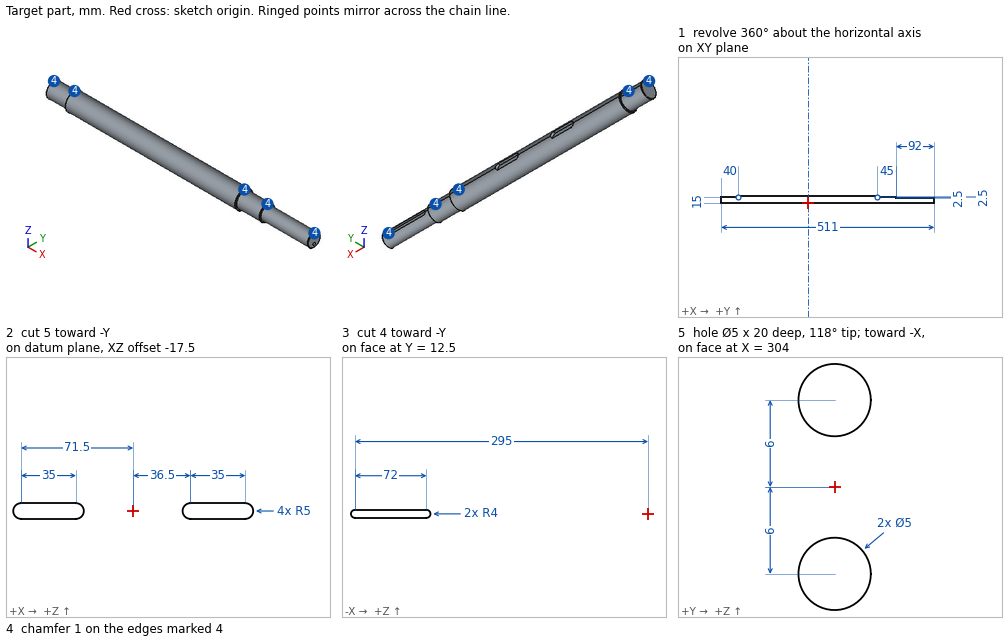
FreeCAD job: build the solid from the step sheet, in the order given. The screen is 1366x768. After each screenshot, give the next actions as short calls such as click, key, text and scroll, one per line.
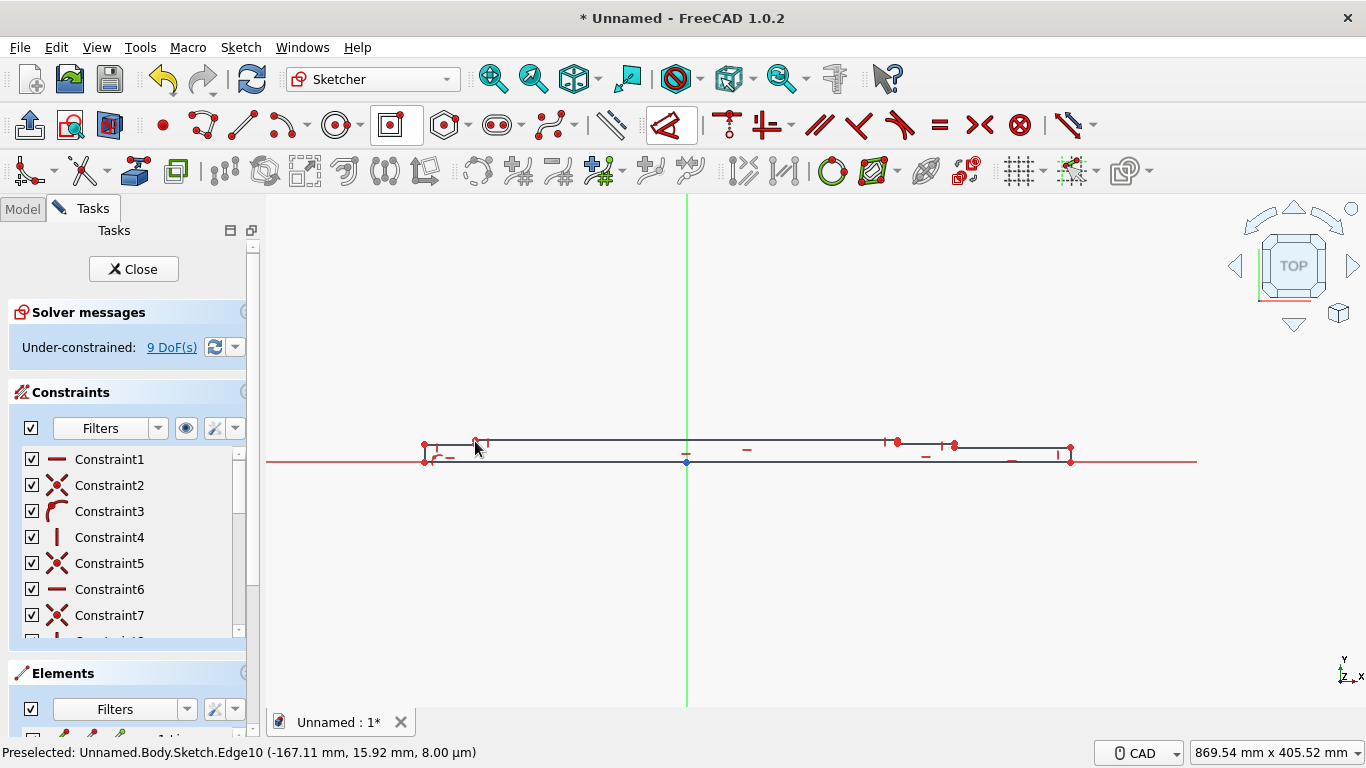
scroll(475, 445, up, 6)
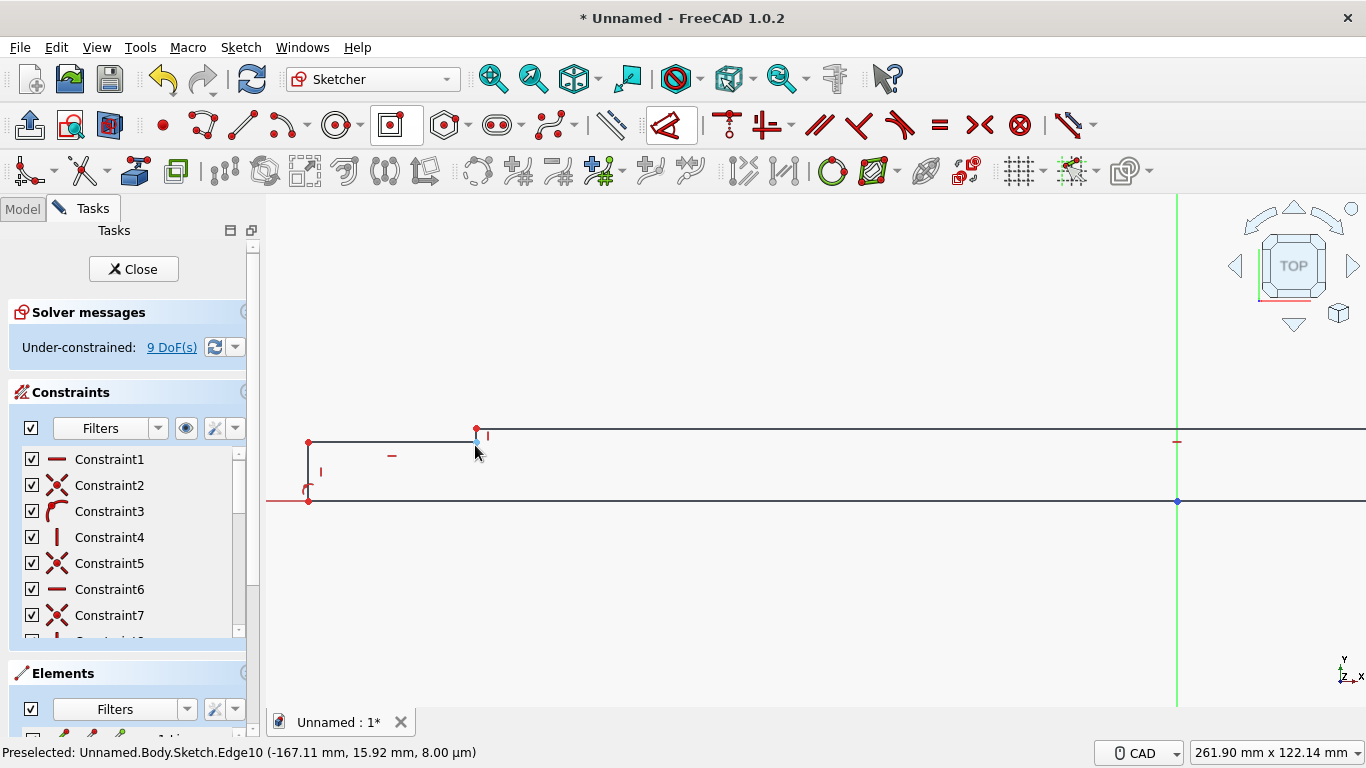
click(476, 442)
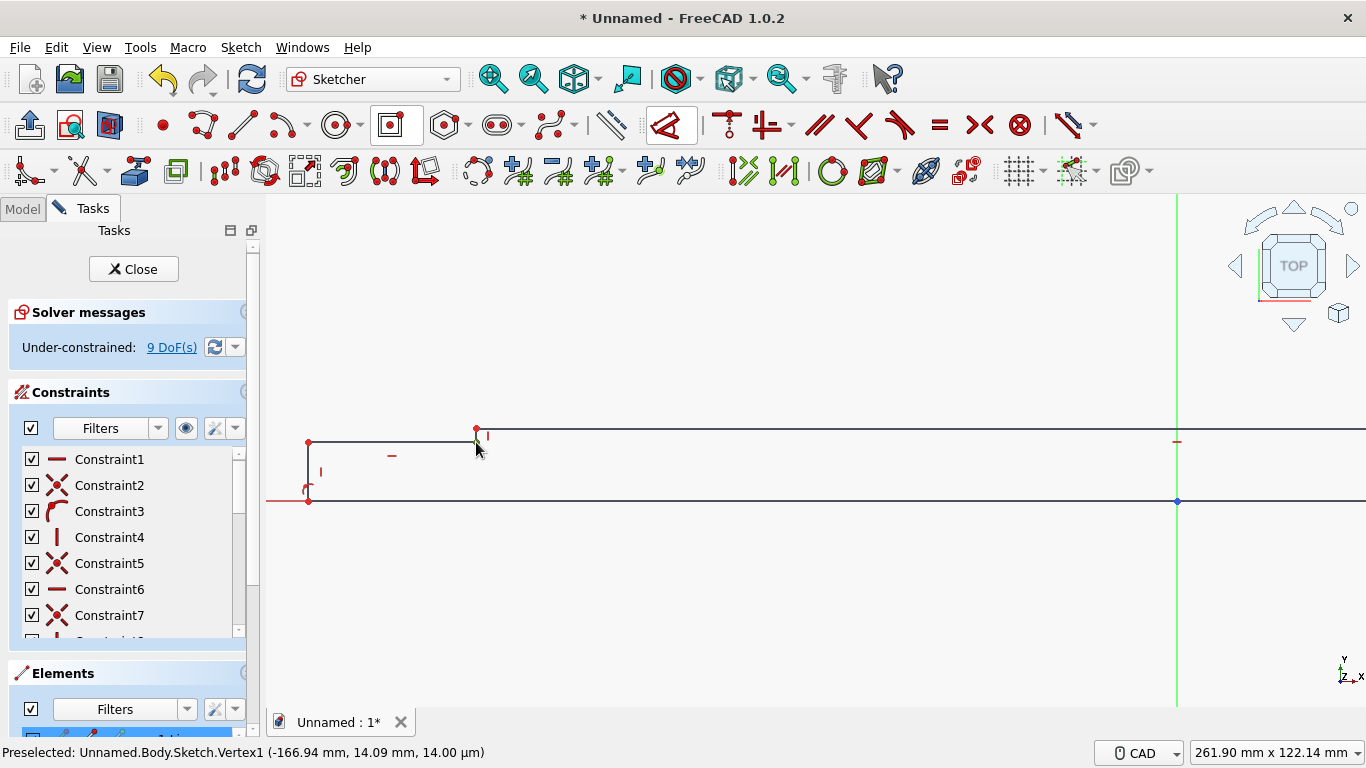
scroll(475, 444, down, 6)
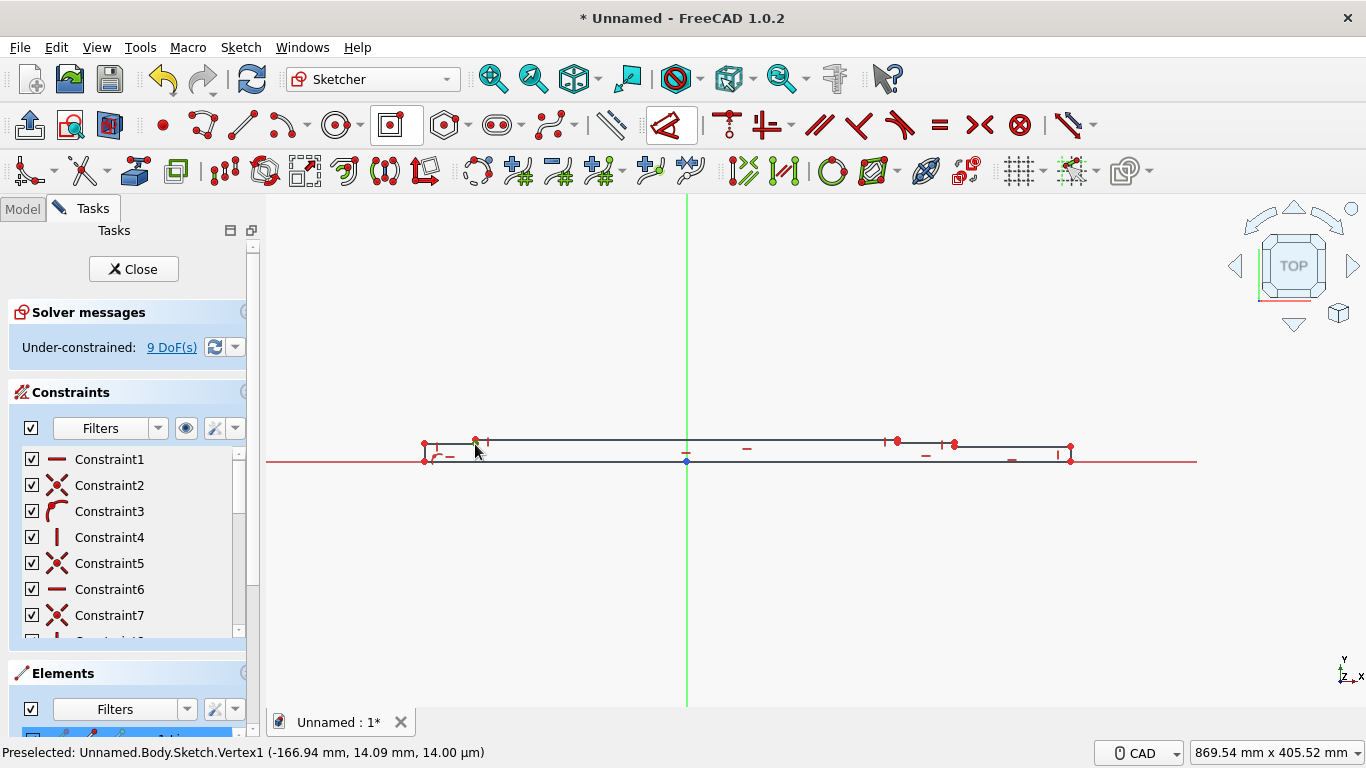
scroll(898, 443, up, 7)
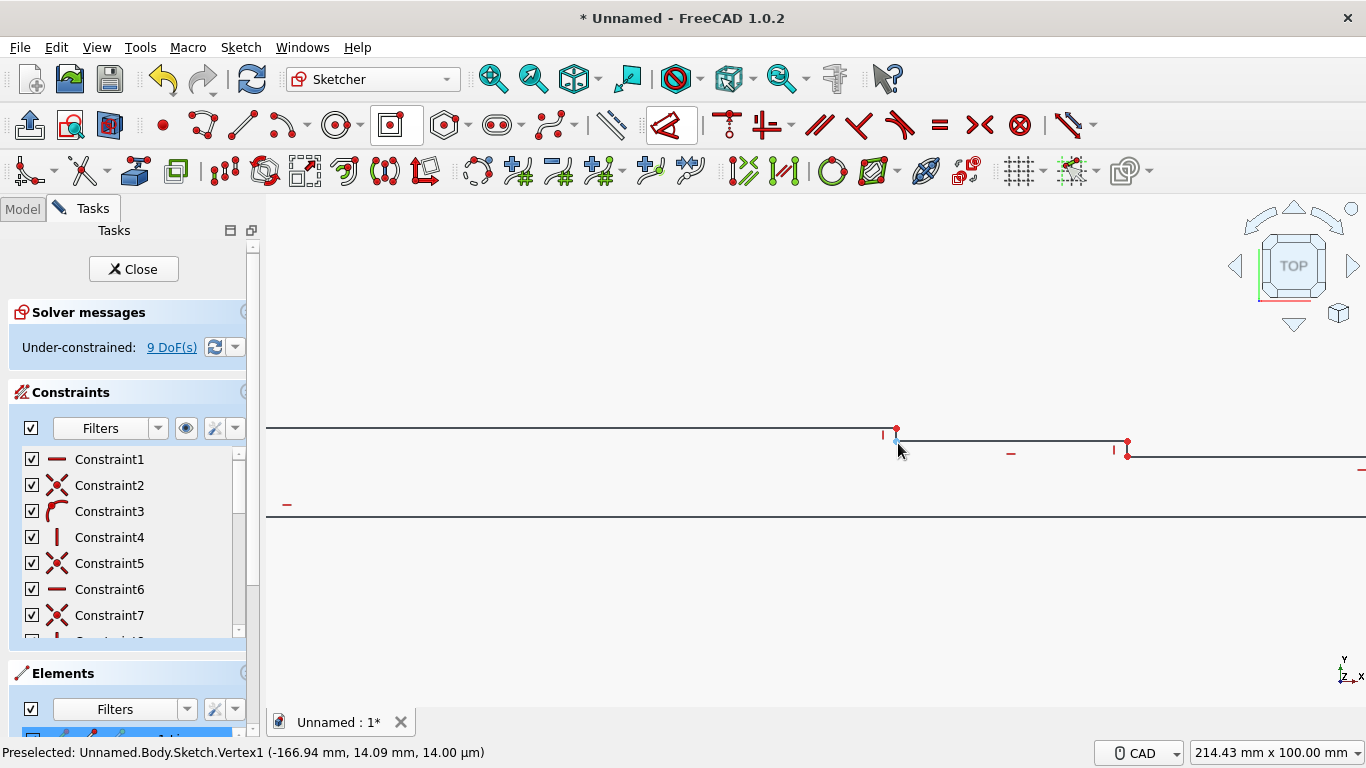
click(896, 441)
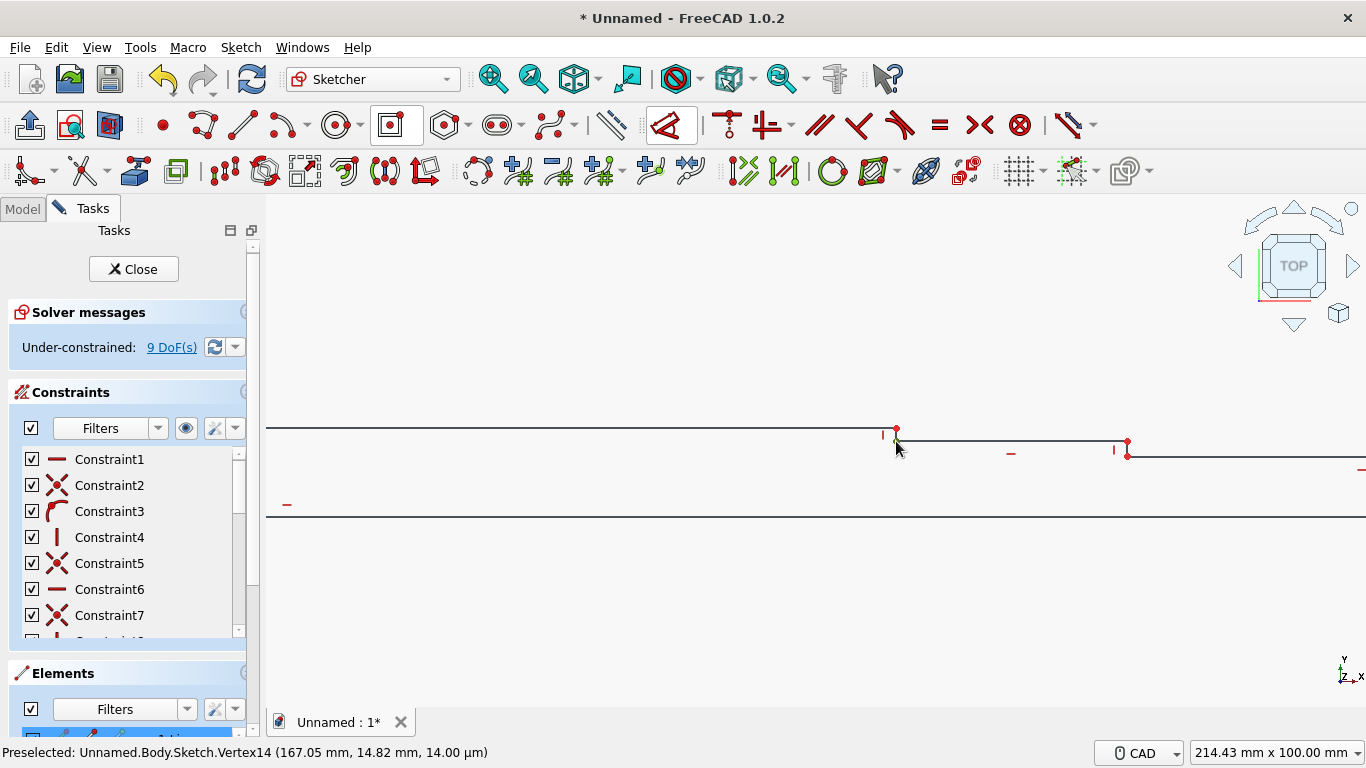
scroll(898, 443, down, 7)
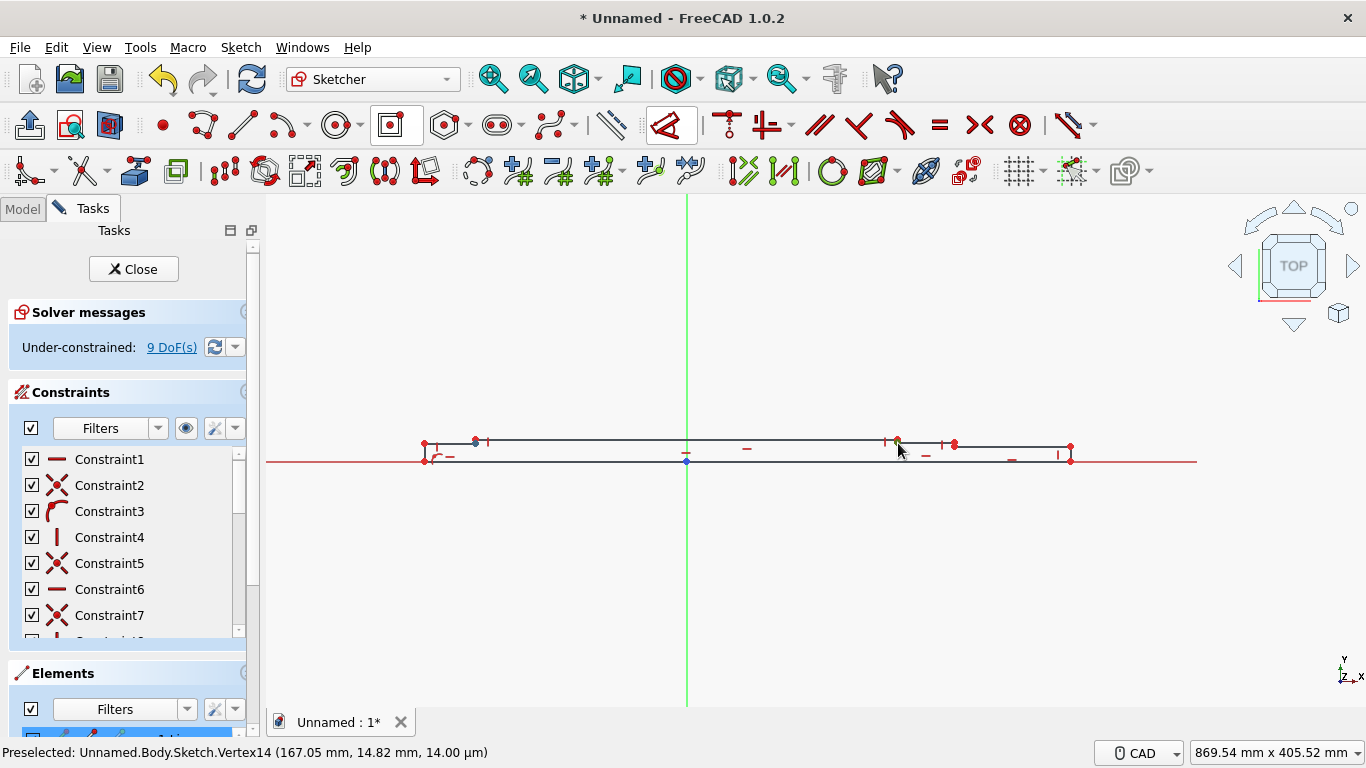
click(687, 646)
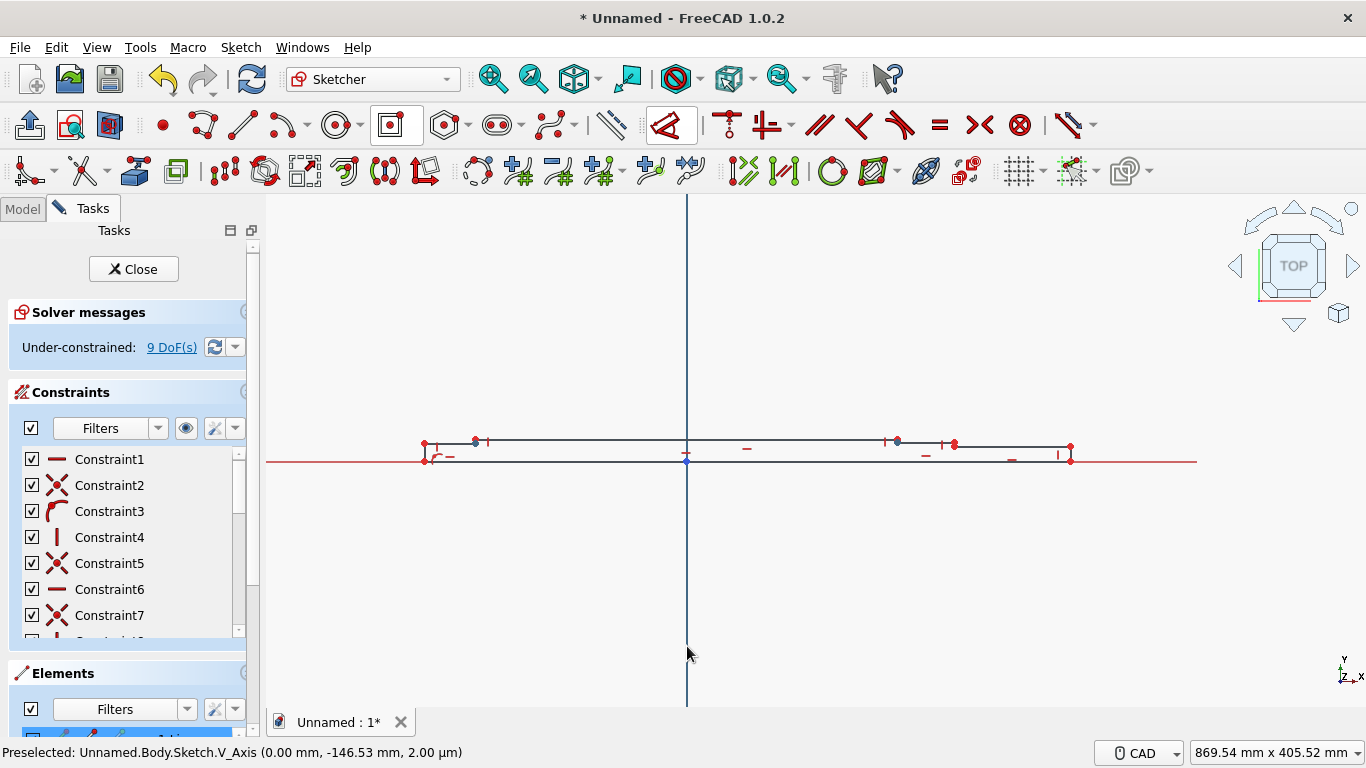
click(980, 126)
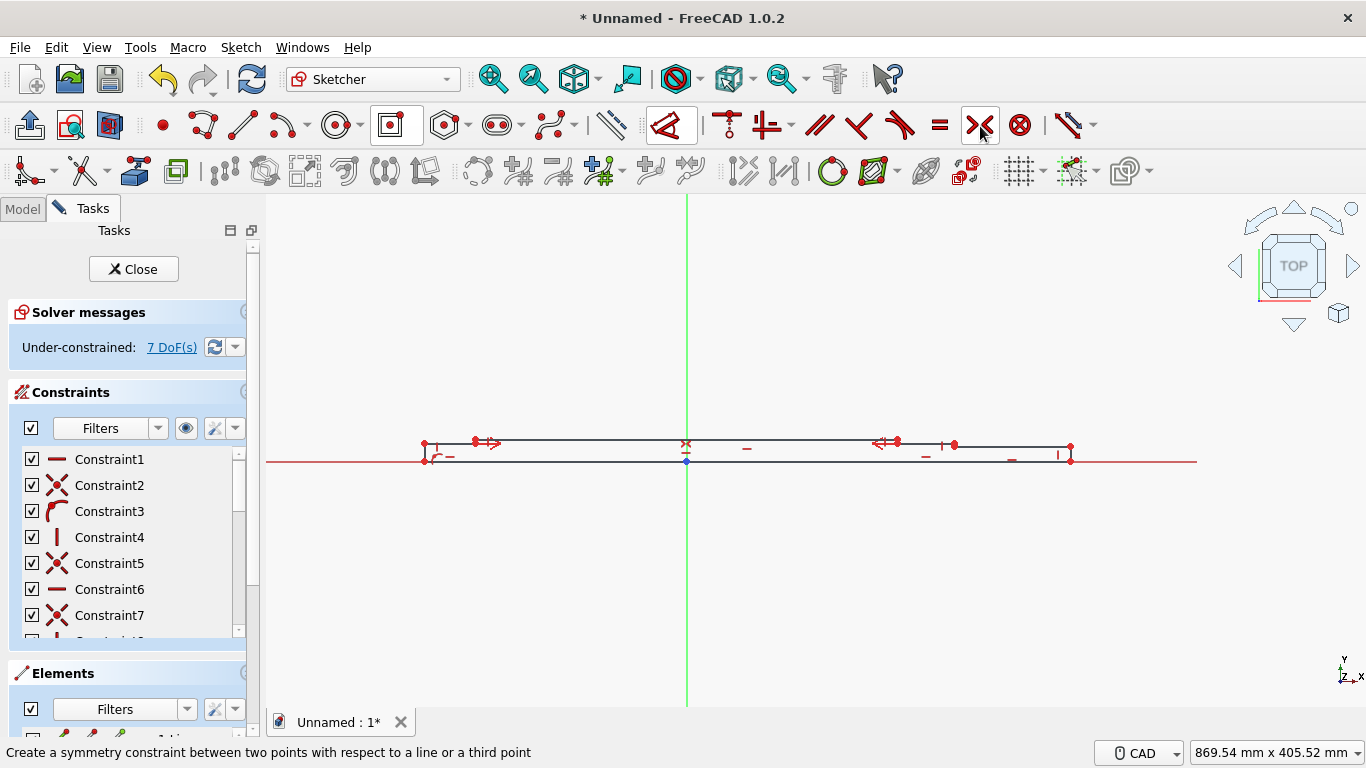
click(460, 444)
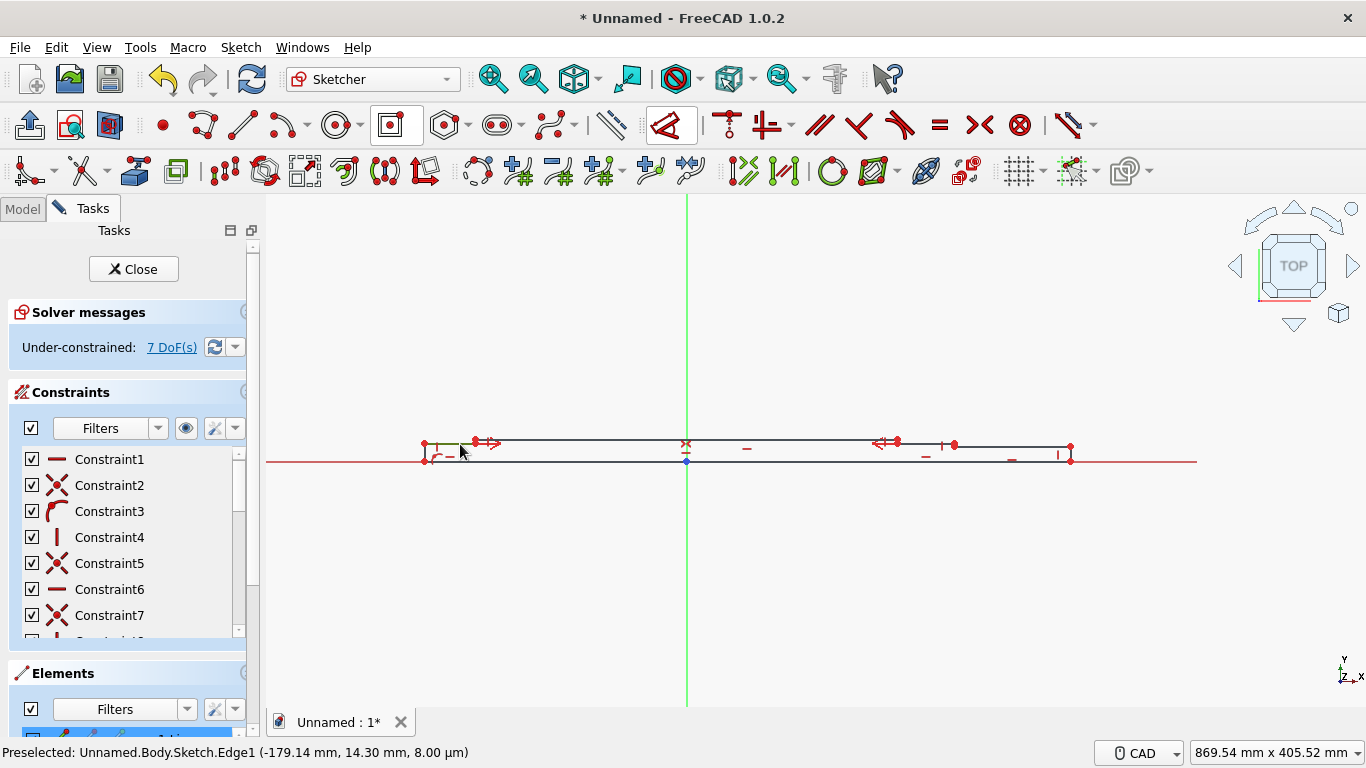
key(l)